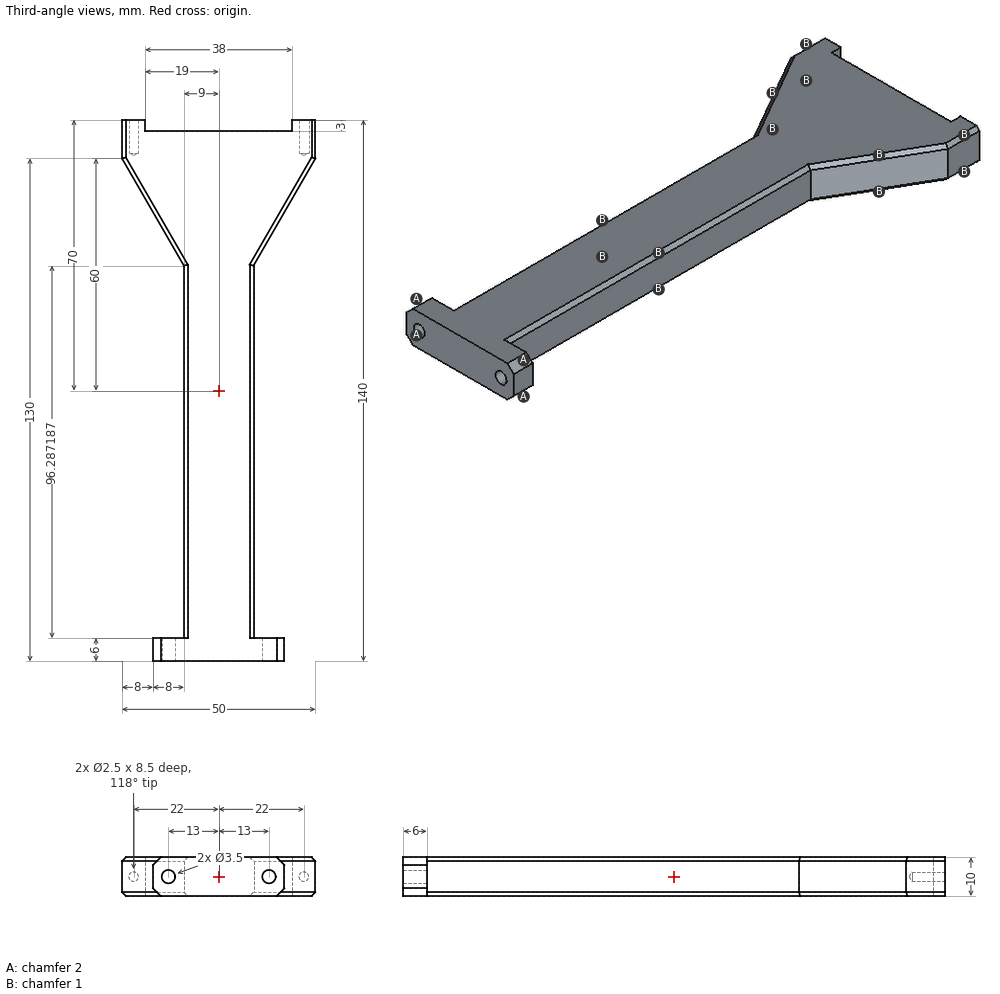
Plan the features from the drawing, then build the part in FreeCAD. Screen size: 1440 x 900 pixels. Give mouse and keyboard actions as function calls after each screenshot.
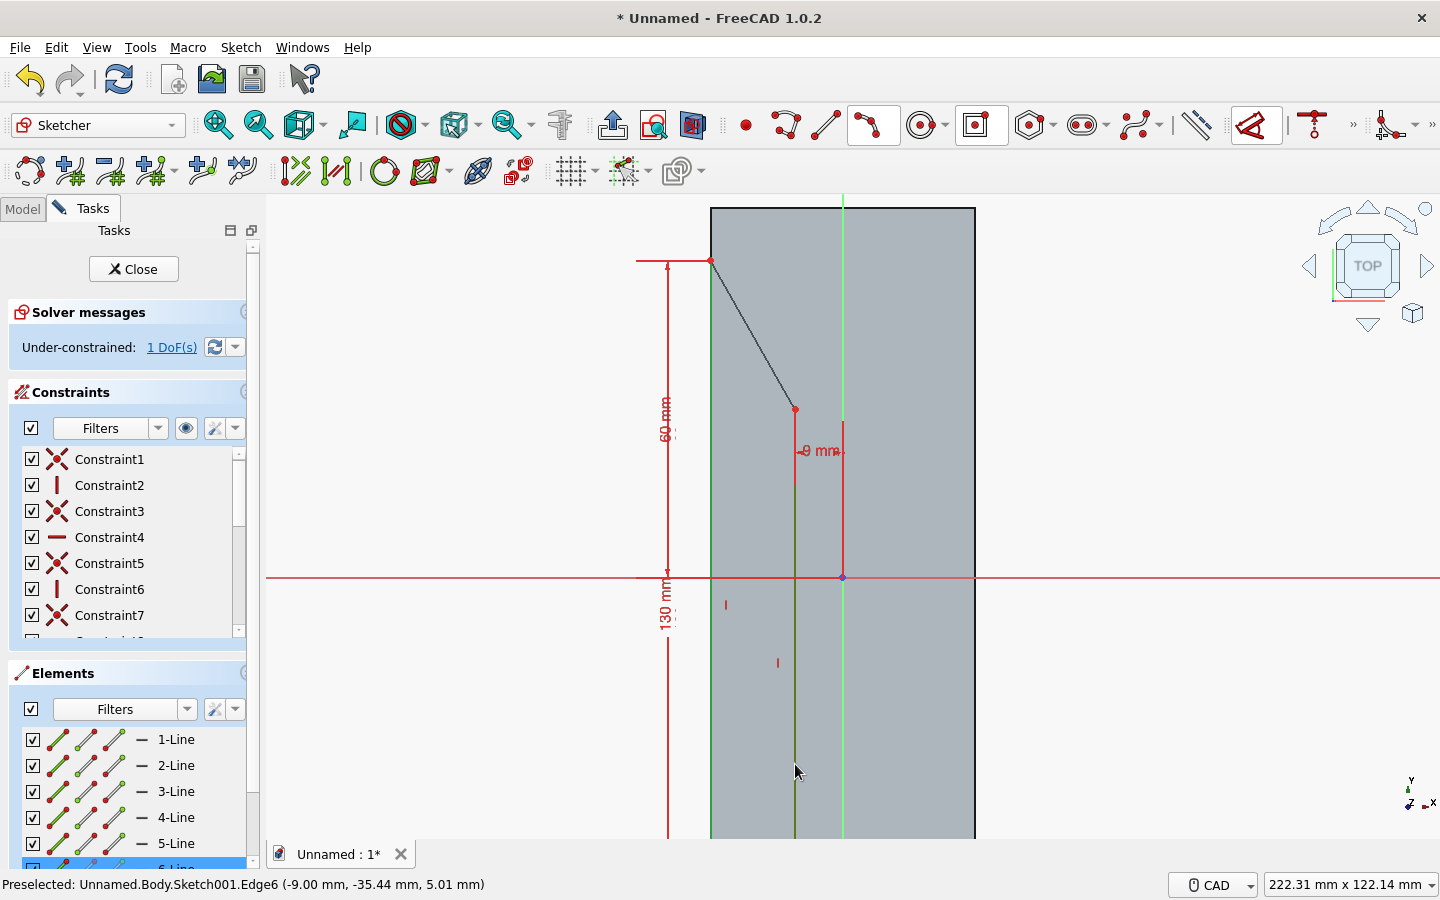
click(1276, 126)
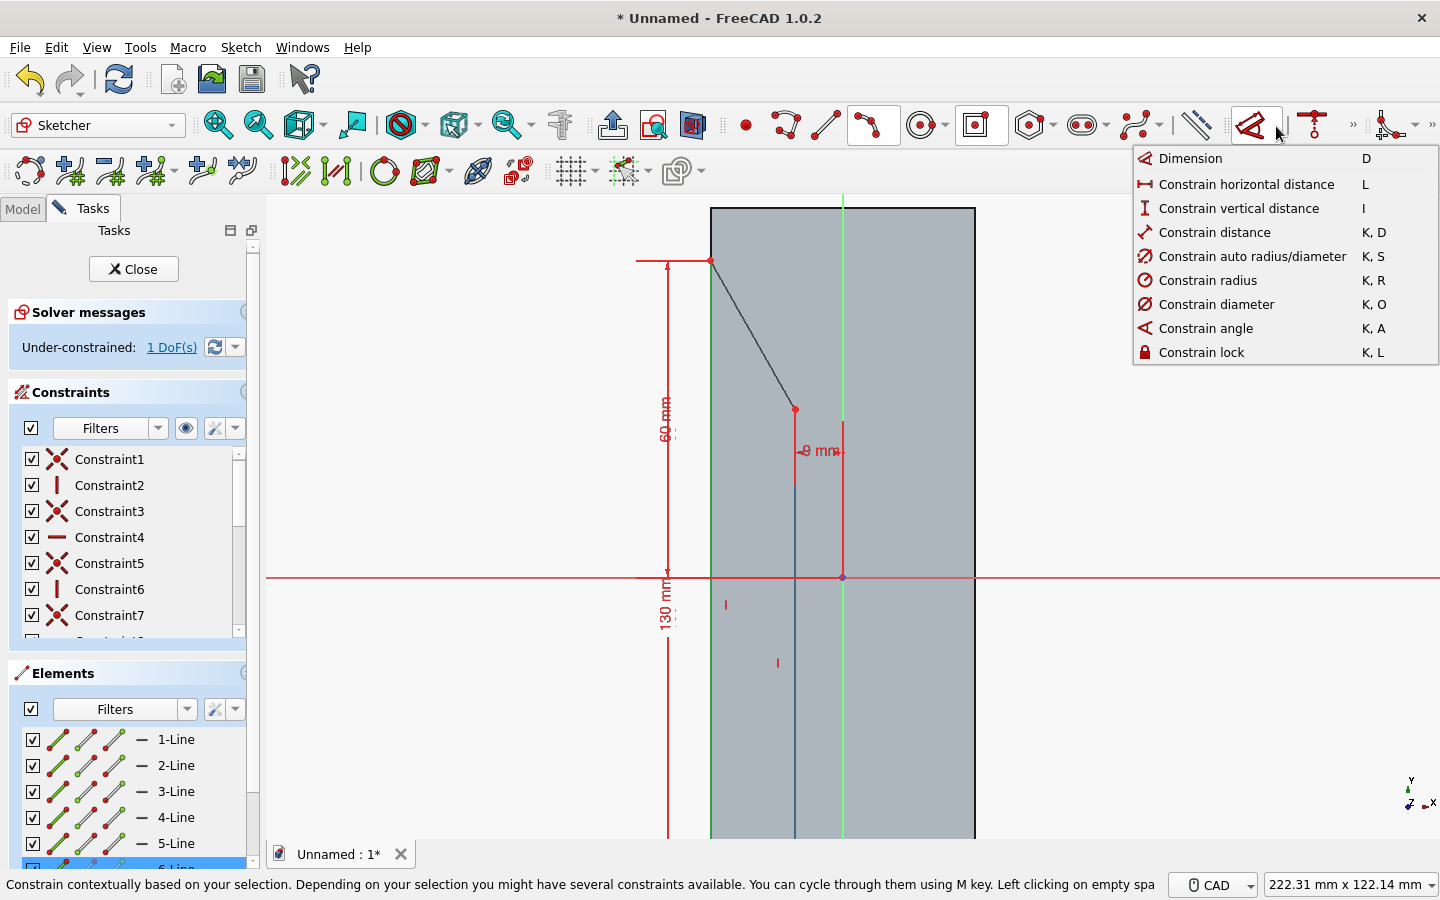
click(1286, 208)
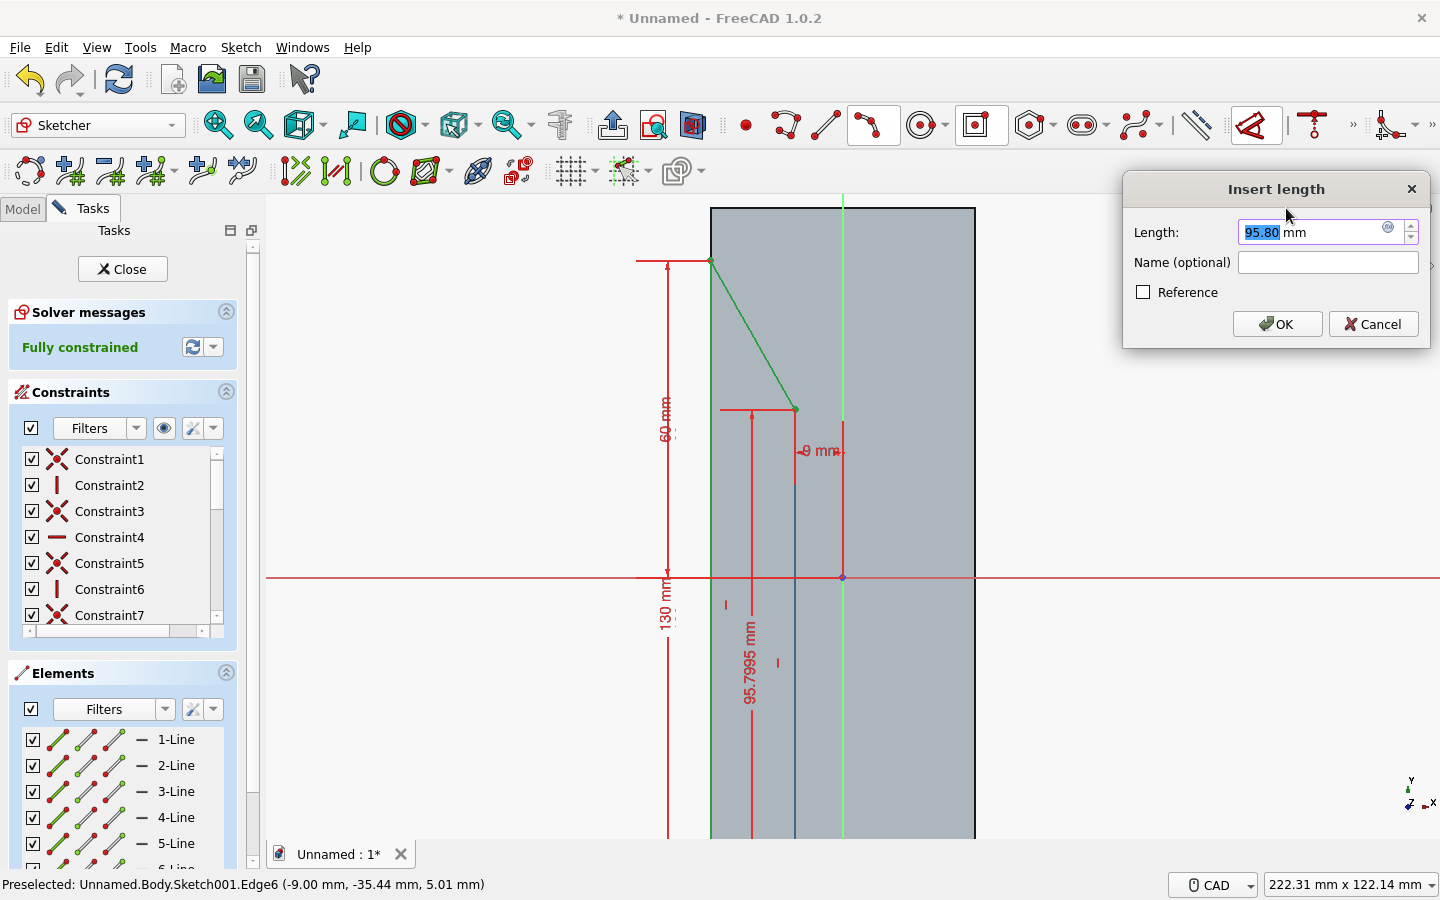
text(96.287187)
key(Return)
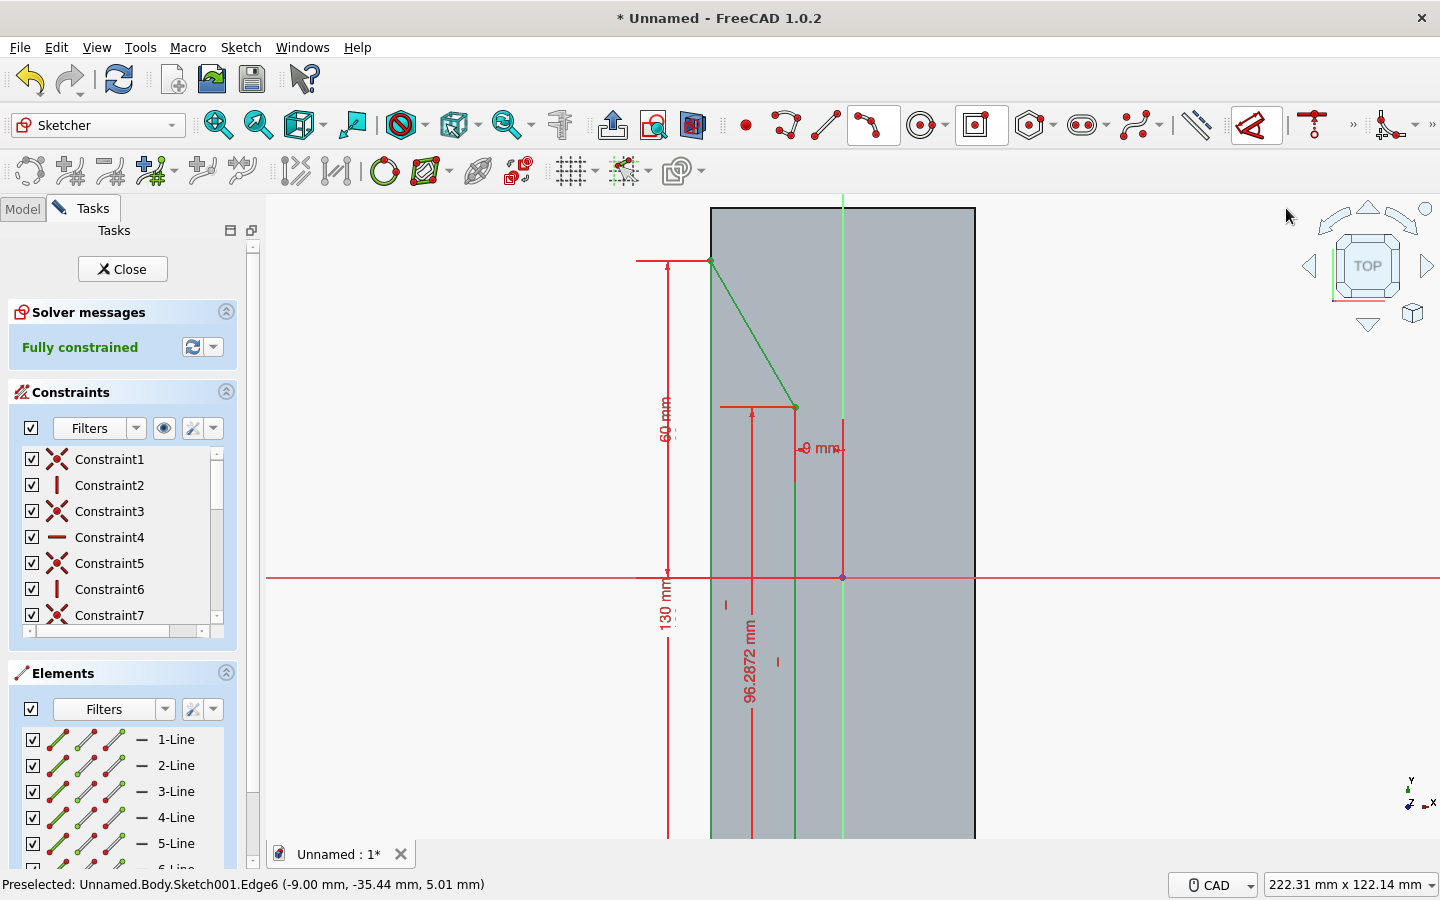
click(123, 269)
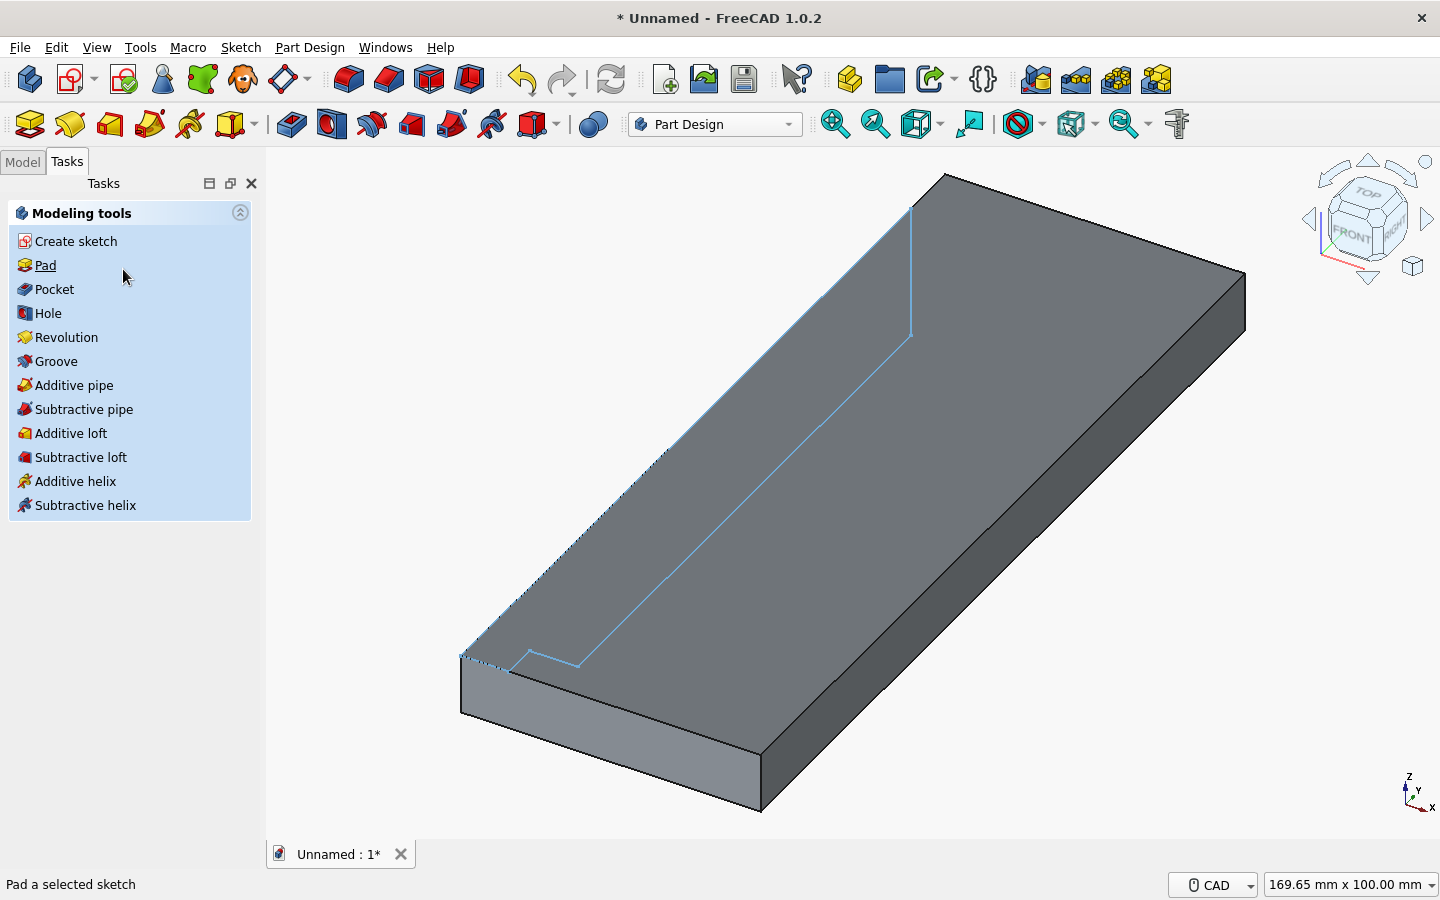
click(292, 124)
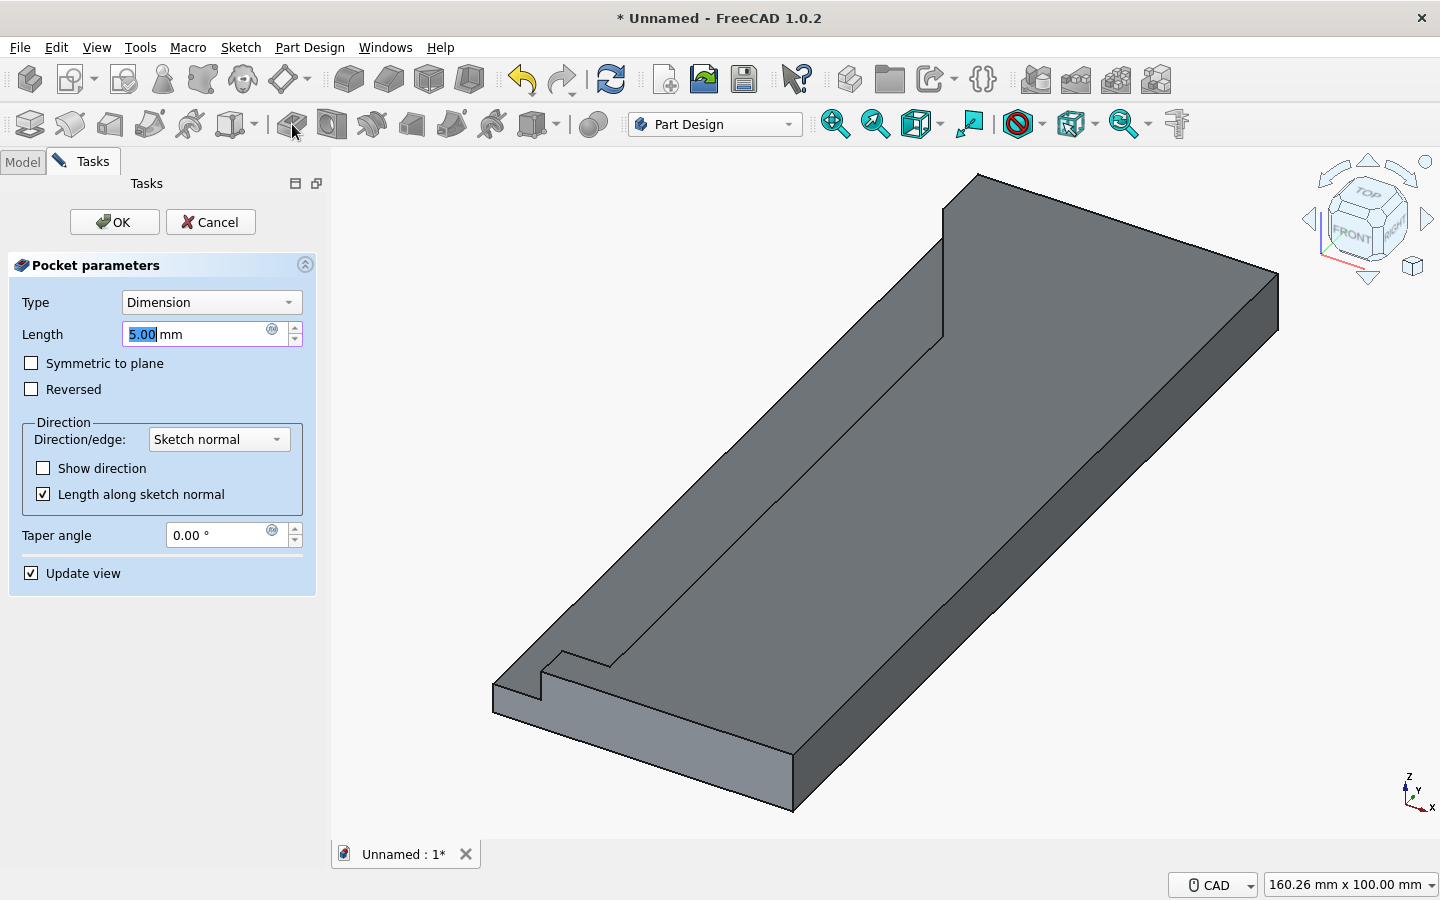
click(212, 302)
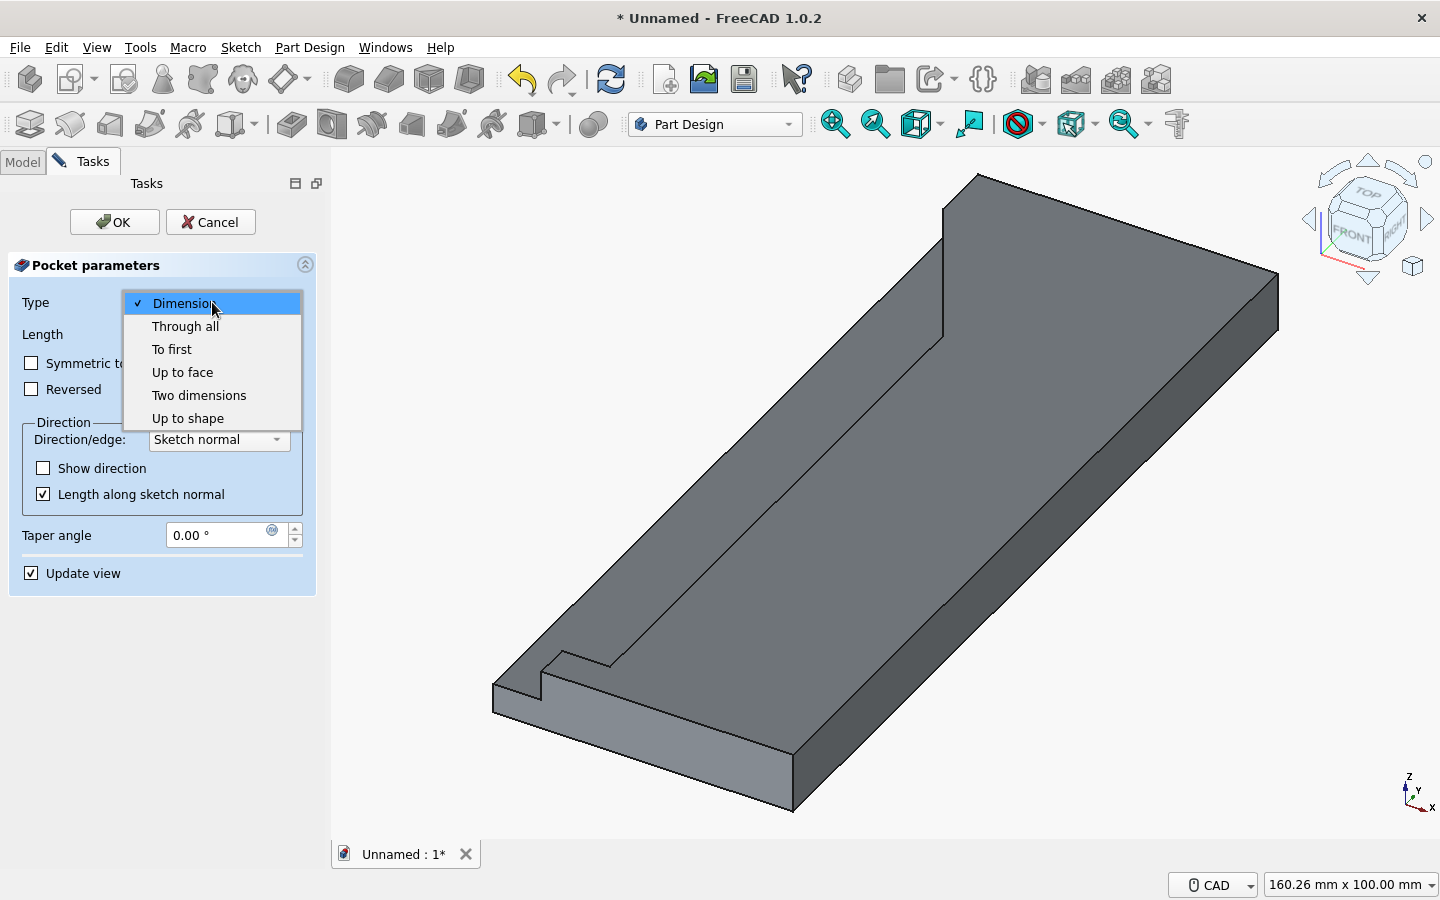
click(212, 326)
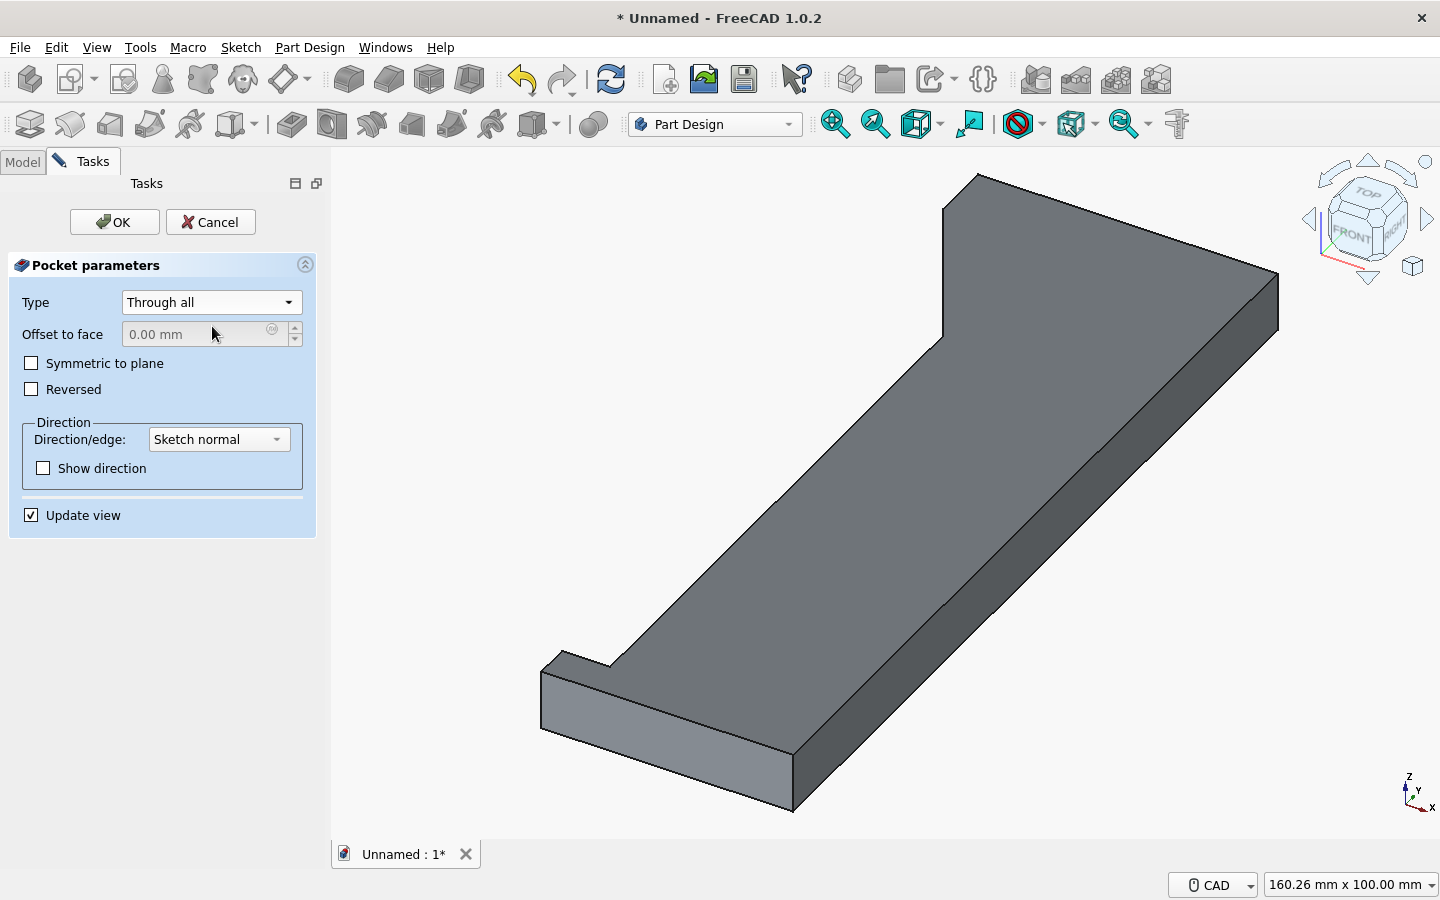
click(115, 222)